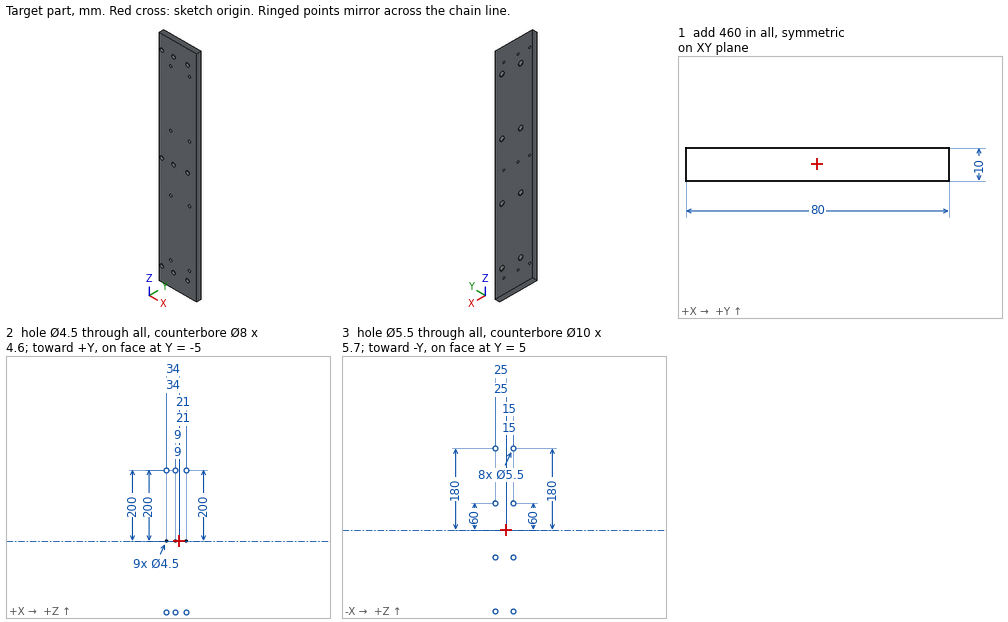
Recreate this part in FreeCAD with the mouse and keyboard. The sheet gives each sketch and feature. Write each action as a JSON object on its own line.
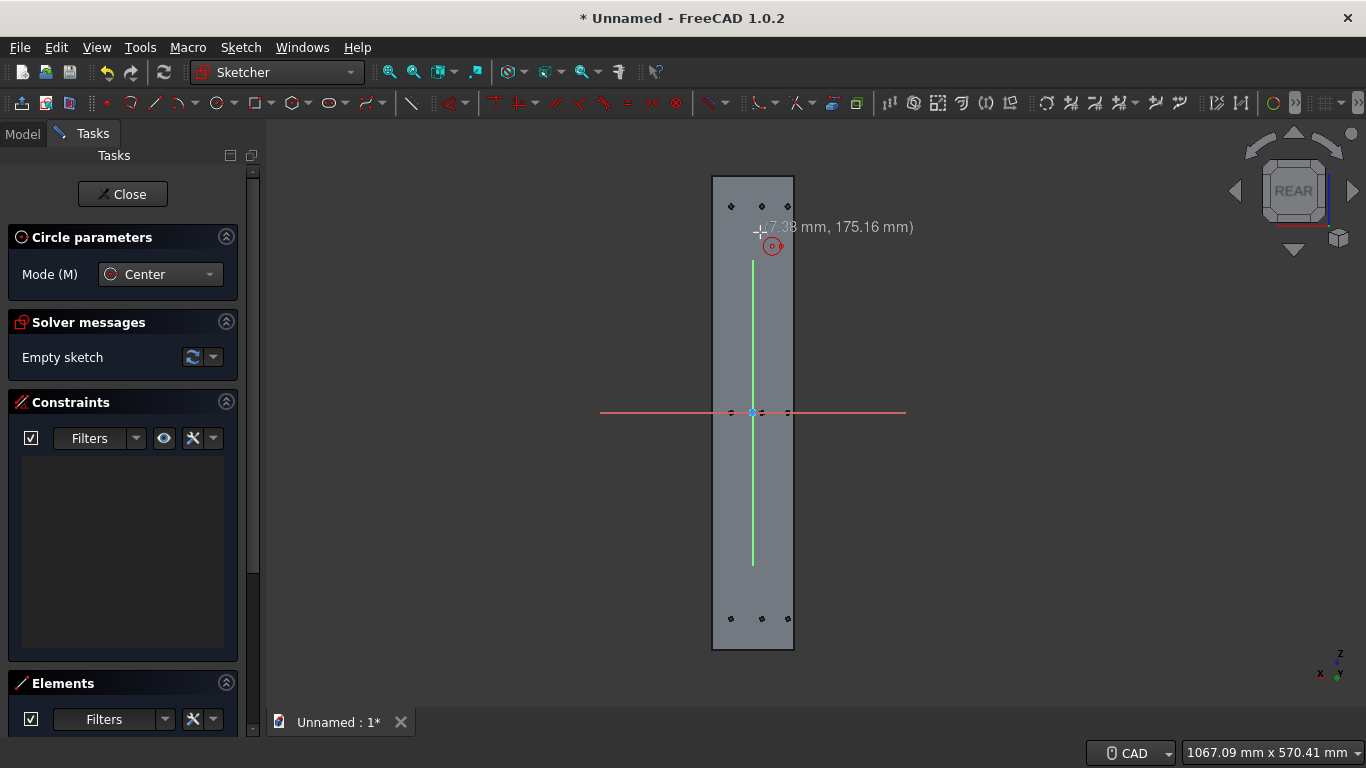
{"action": "left_click", "coordinate": [768, 227]}
{"action": "mouse_move", "coordinate": [770, 225]}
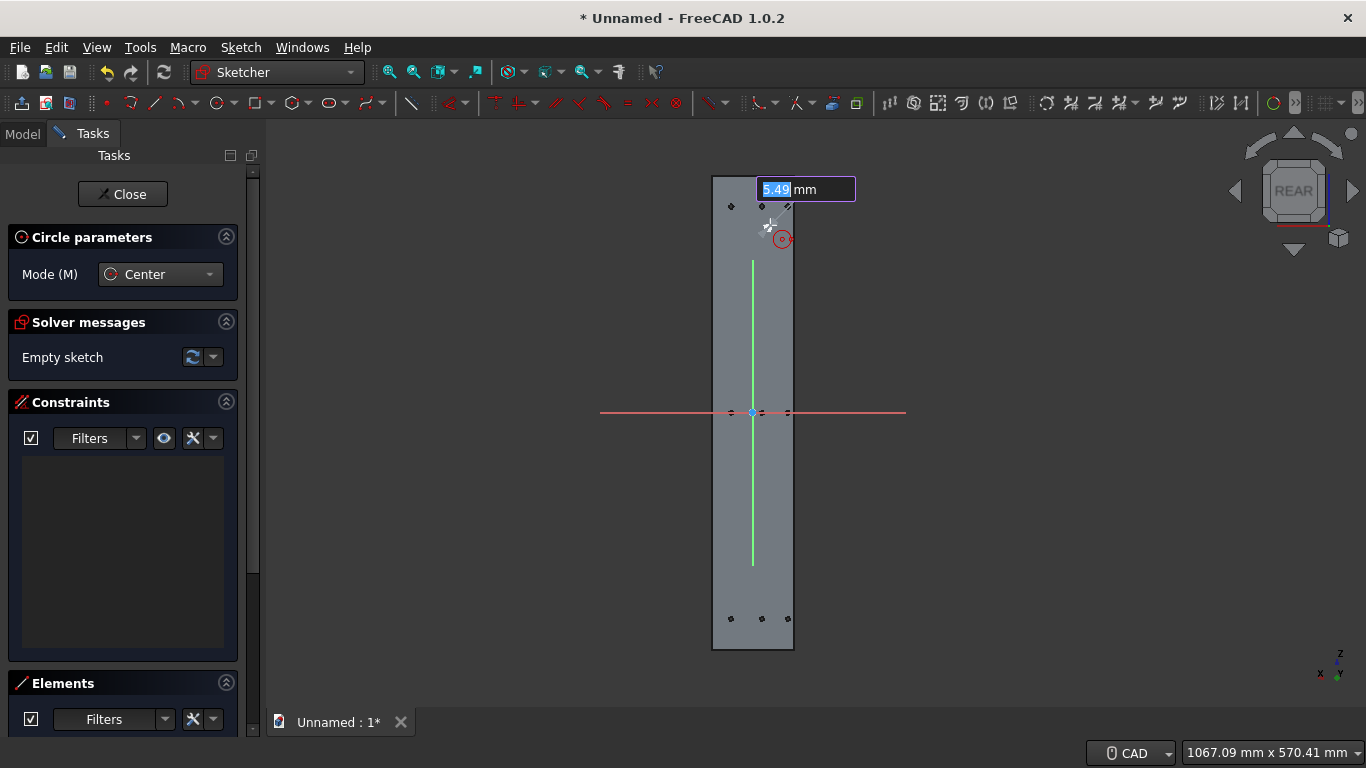
{"action": "type", "text": "5.5"}
{"action": "key", "text": "Return"}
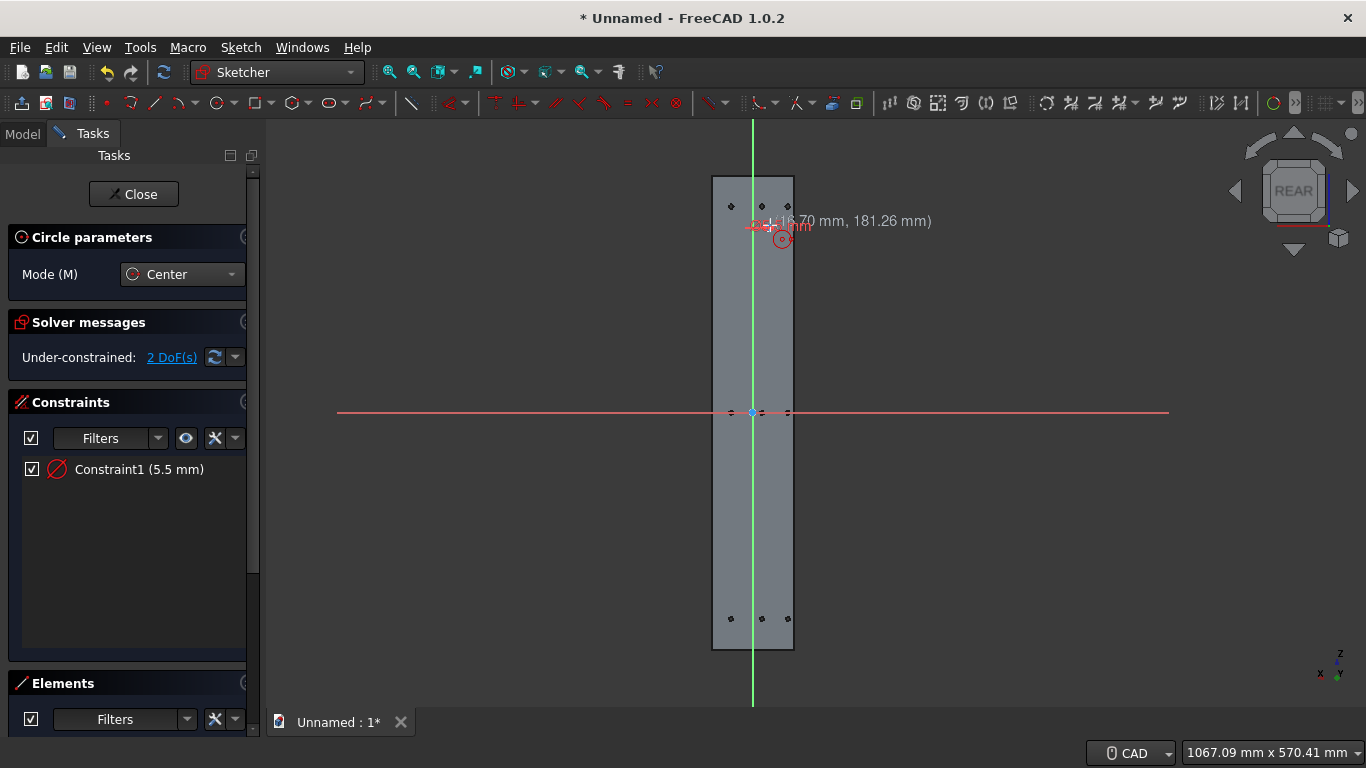
{"action": "scroll", "coordinate": [727, 227], "scroll_direction": "up", "scroll_amount": 11}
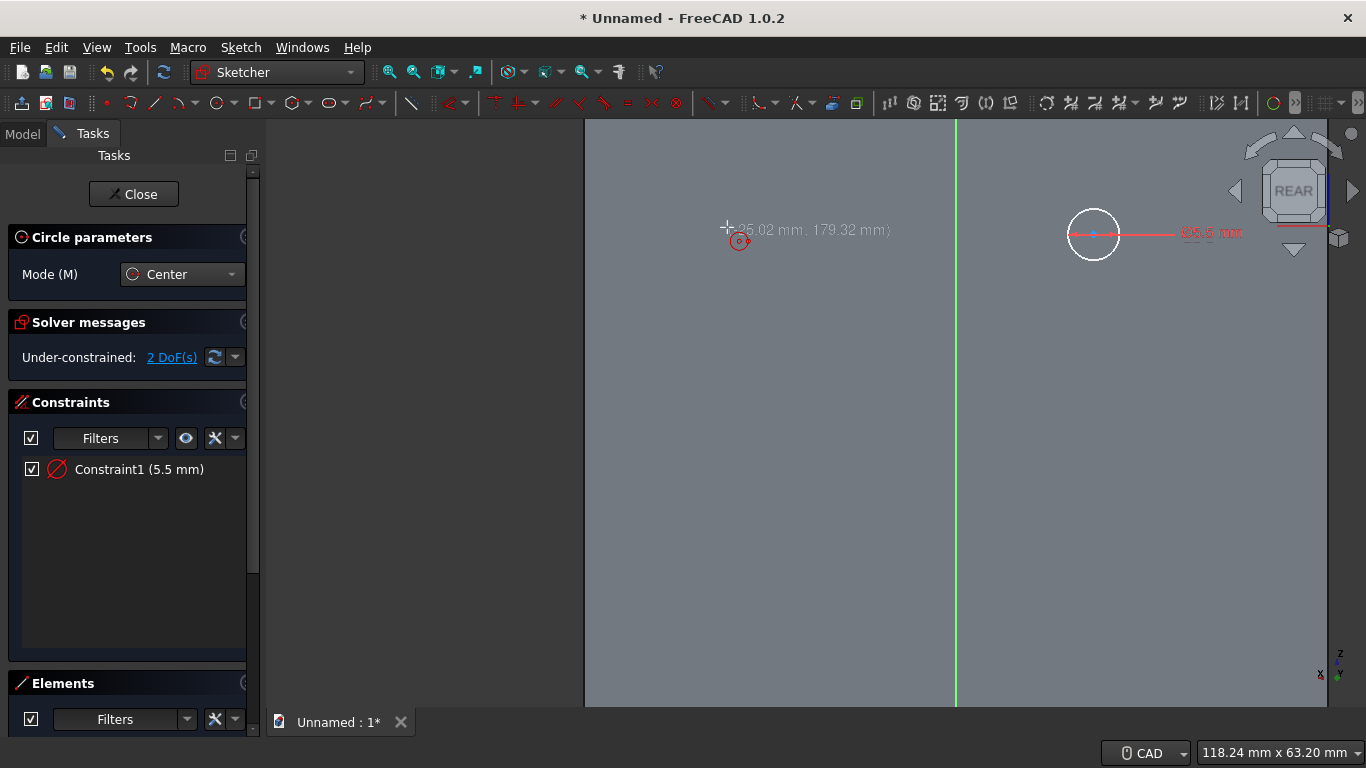
{"action": "scroll", "coordinate": [727, 227], "scroll_direction": "down", "scroll_amount": 11}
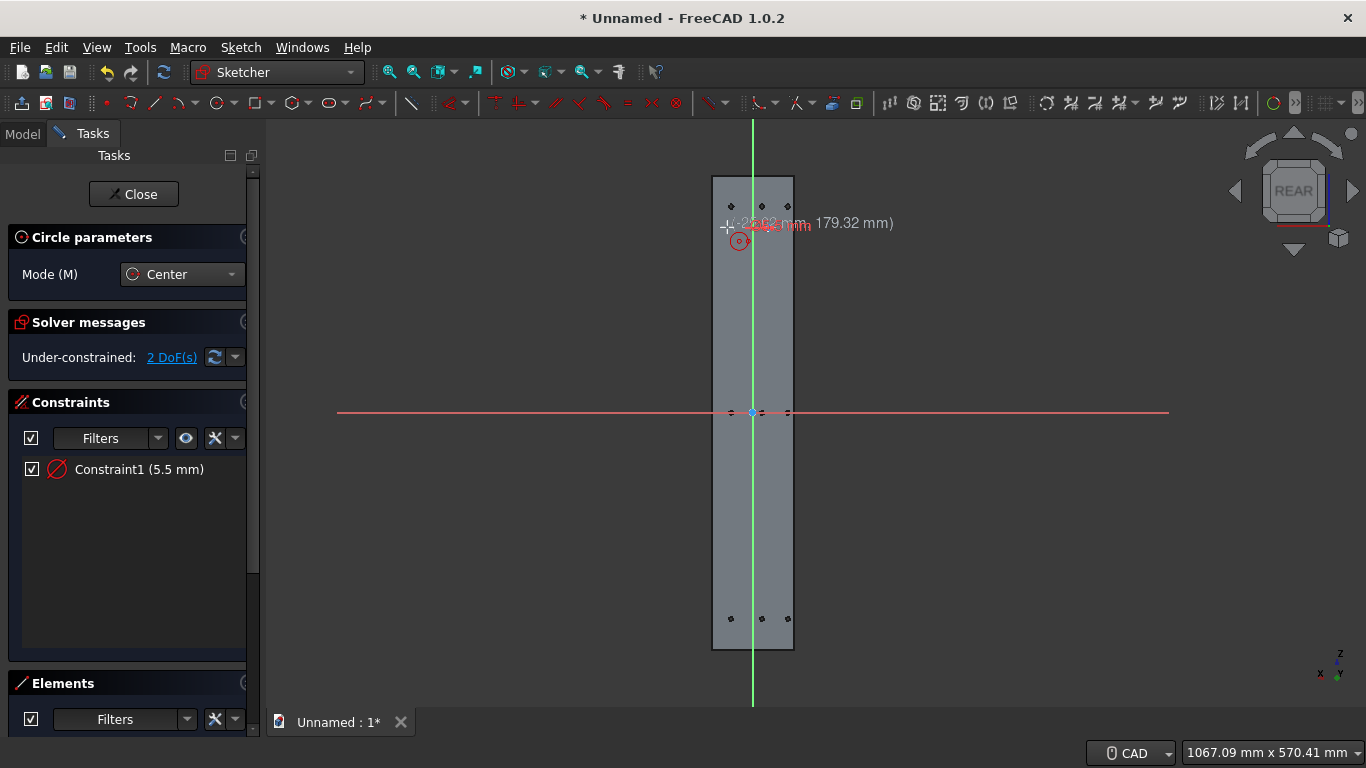
{"action": "left_click", "coordinate": [727, 227]}
{"action": "mouse_move", "coordinate": [729, 225]}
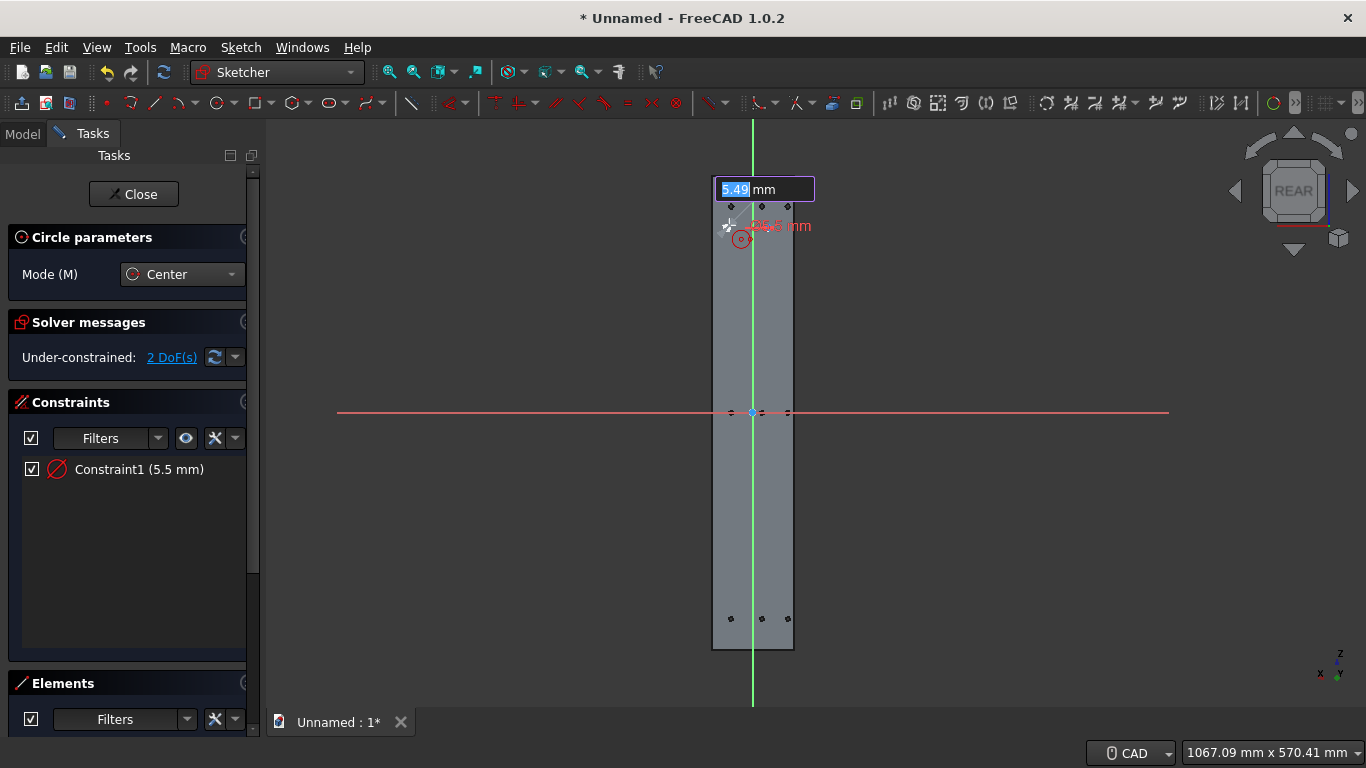
{"action": "type", "text": "5.5"}
{"action": "key", "text": "Return"}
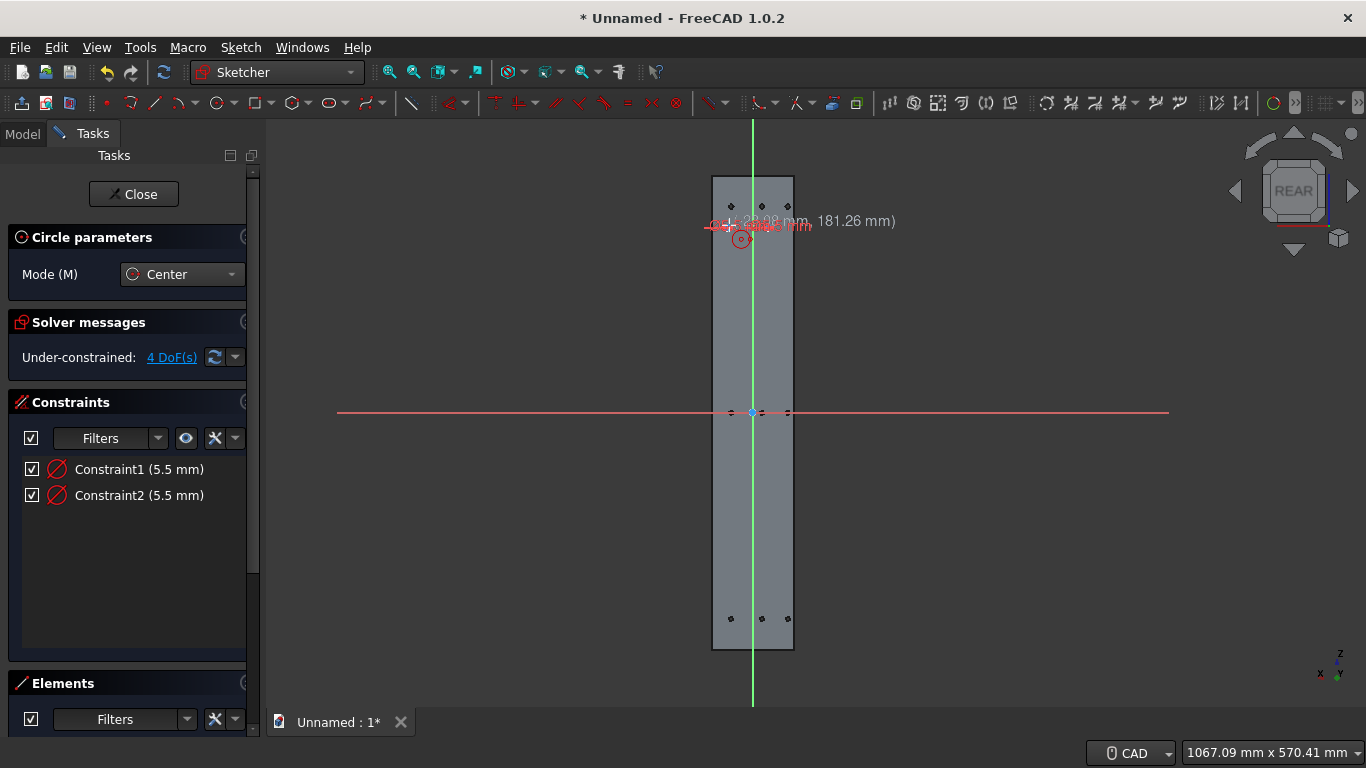
{"action": "scroll", "coordinate": [768, 351], "scroll_direction": "up", "scroll_amount": 11}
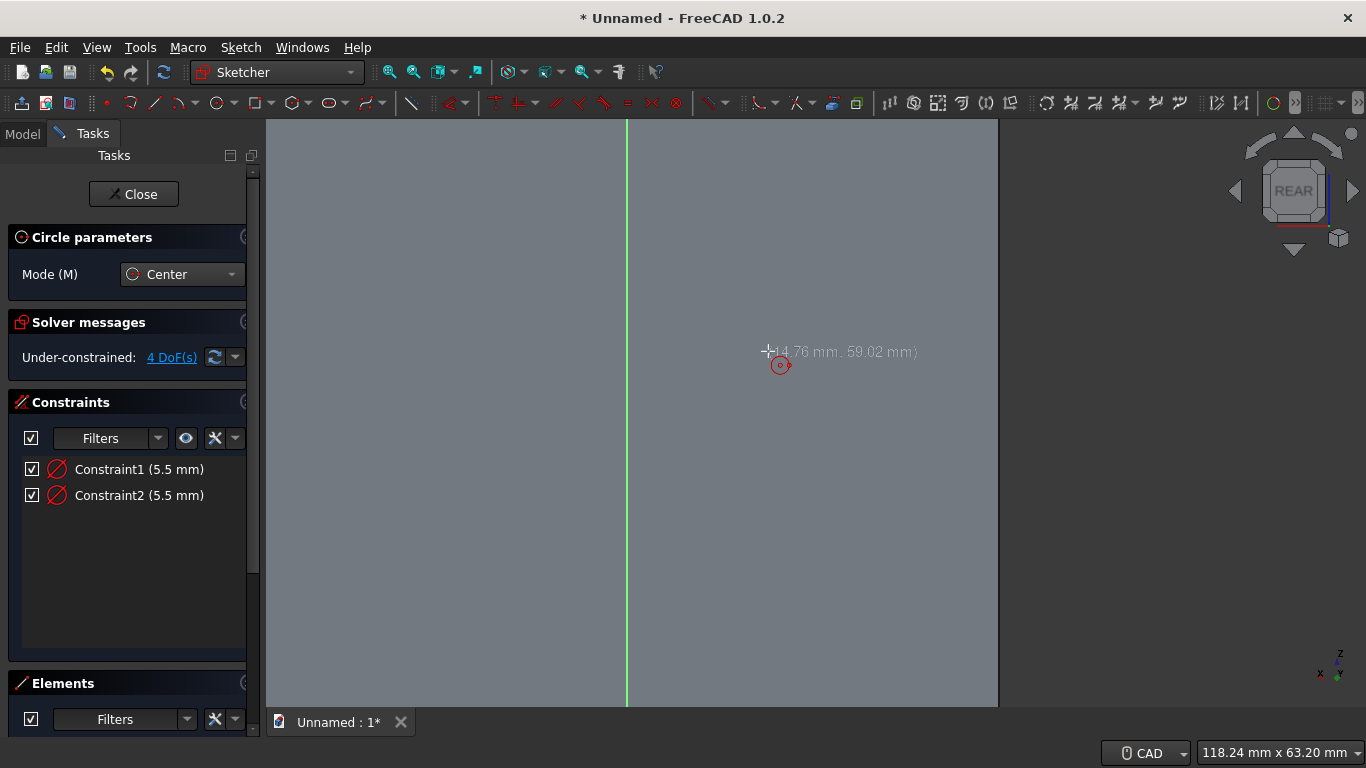
{"action": "scroll", "coordinate": [768, 352], "scroll_direction": "down", "scroll_amount": 11}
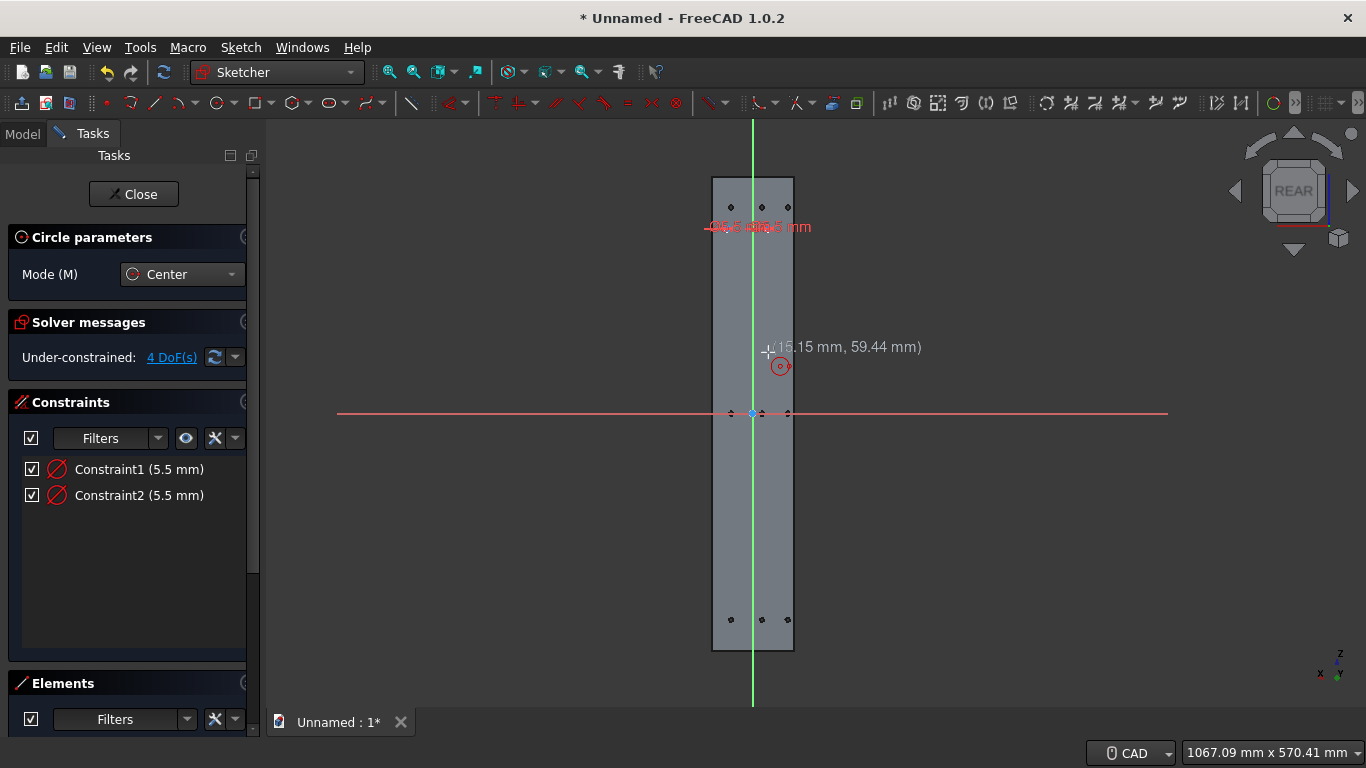
{"action": "left_click", "coordinate": [768, 352]}
{"action": "mouse_move", "coordinate": [770, 350]}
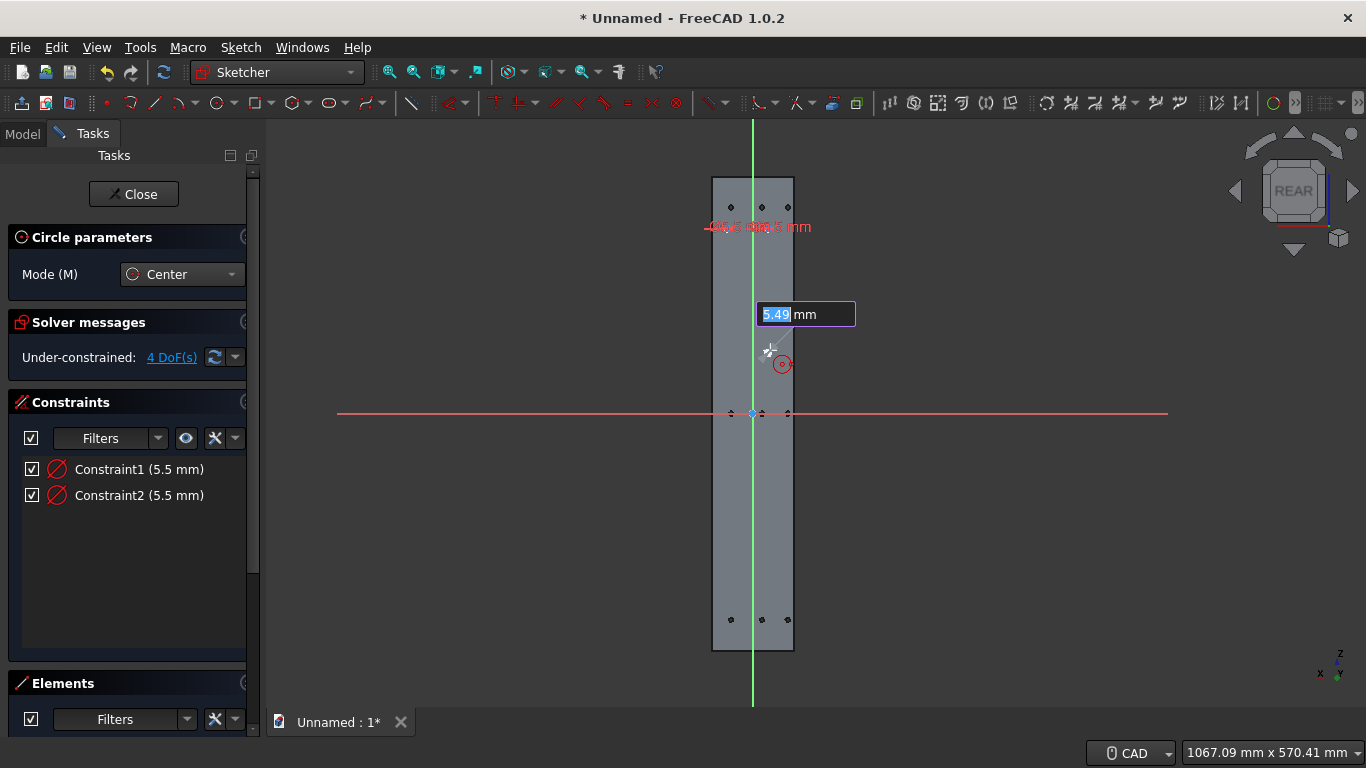
{"action": "type", "text": "5.5"}
{"action": "key", "text": "Return"}